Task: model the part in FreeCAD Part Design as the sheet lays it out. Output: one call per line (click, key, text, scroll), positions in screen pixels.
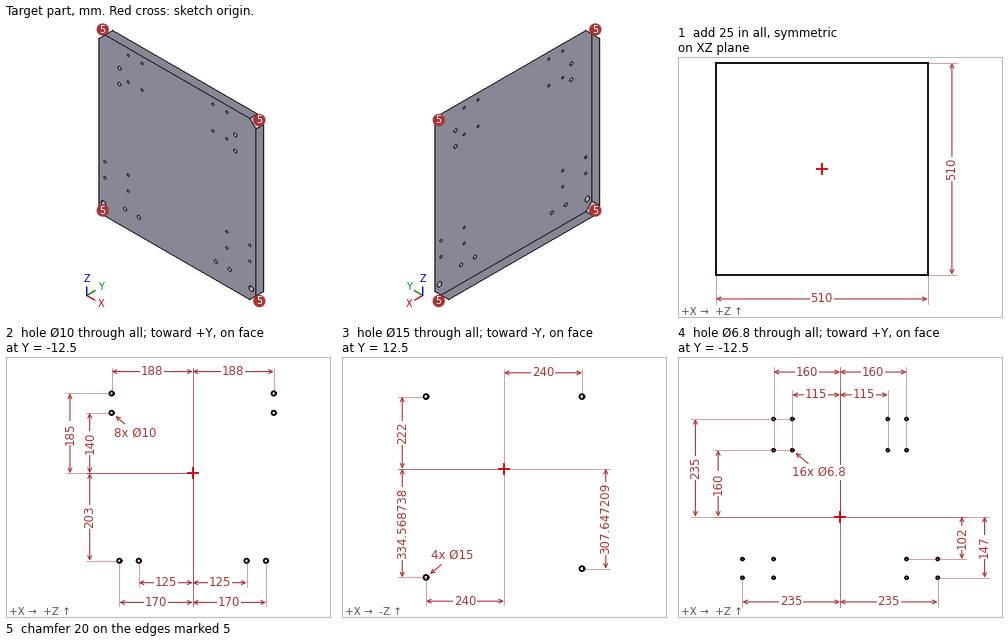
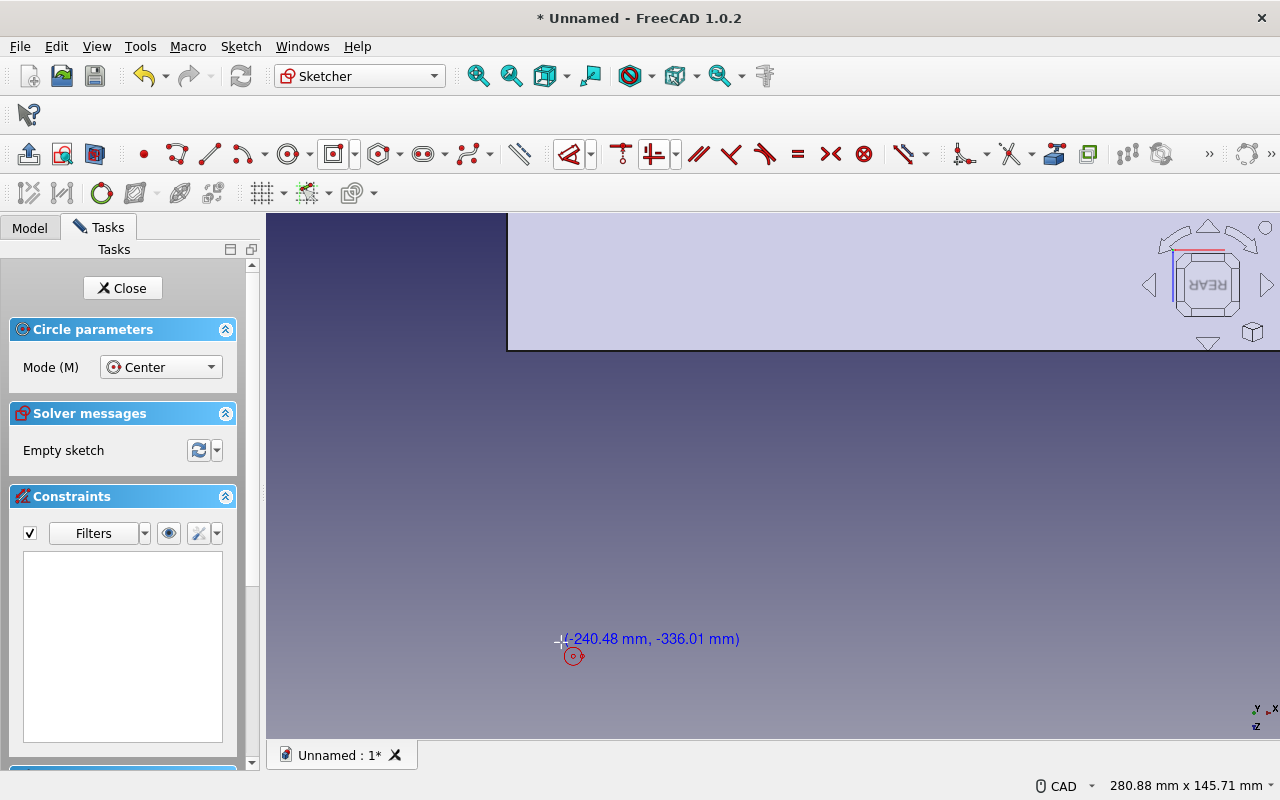
scroll(561, 643, down, 9)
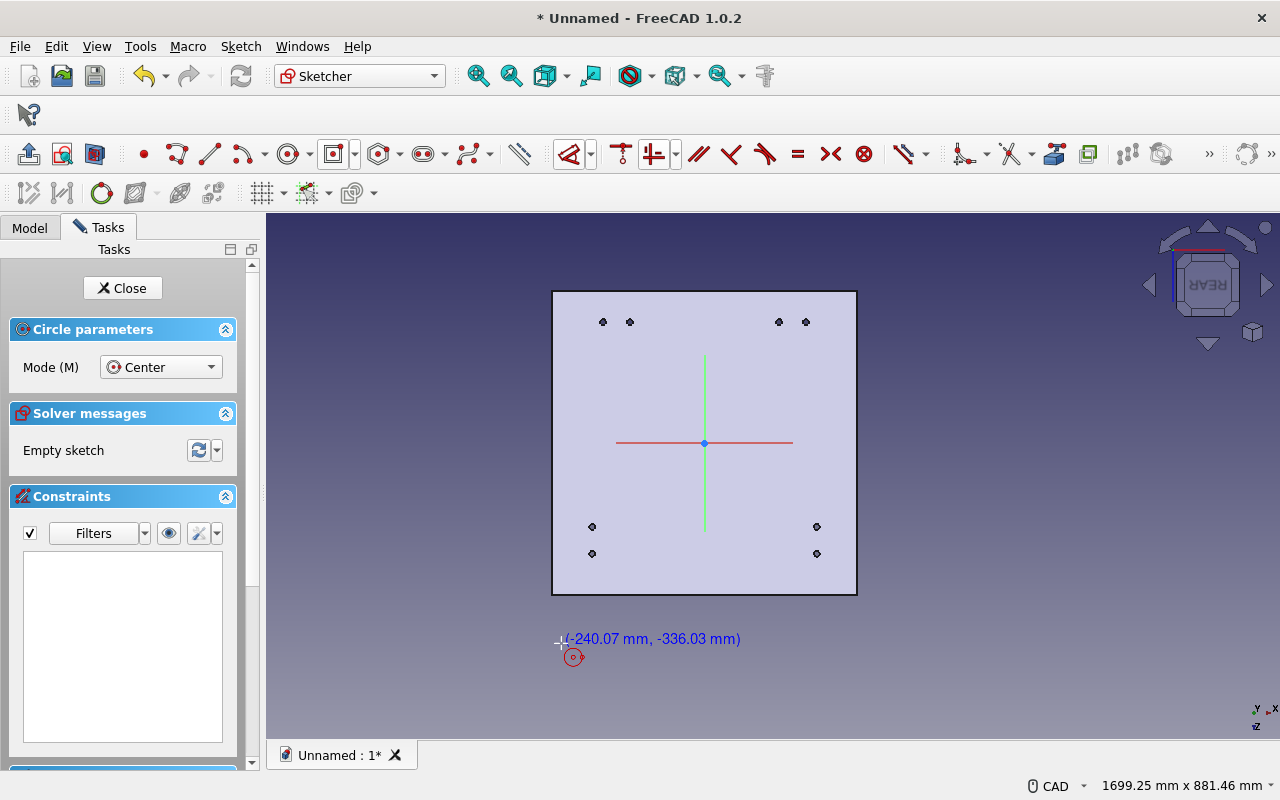
click(561, 643)
move(564, 640)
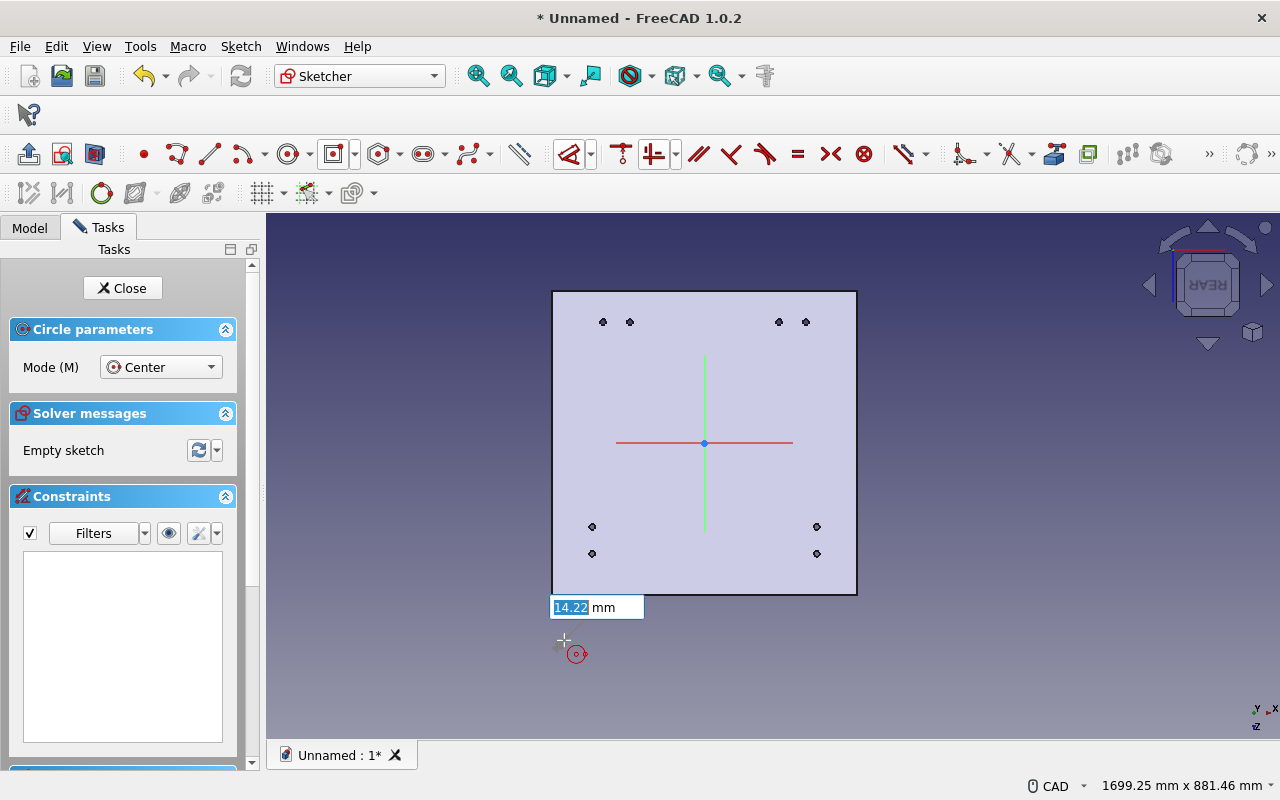
text(15)
key(Return)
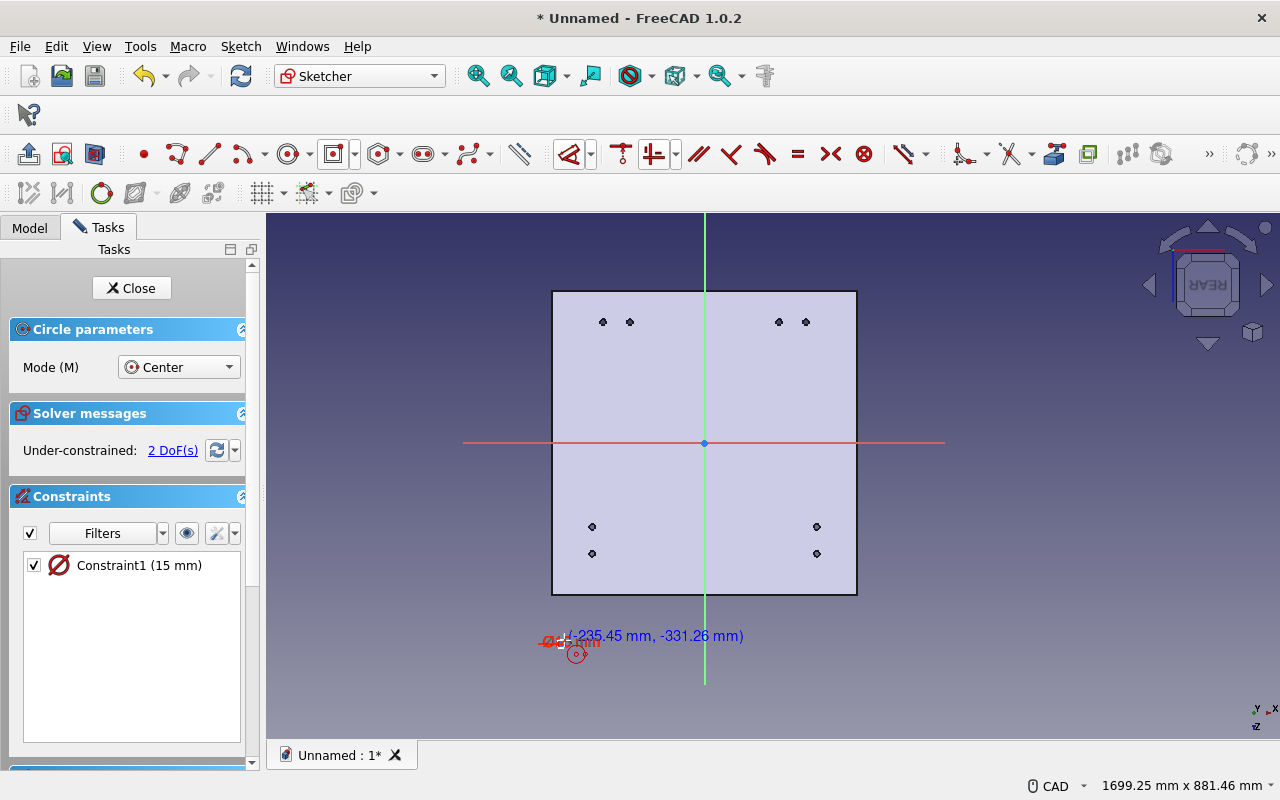
scroll(561, 311, up, 9)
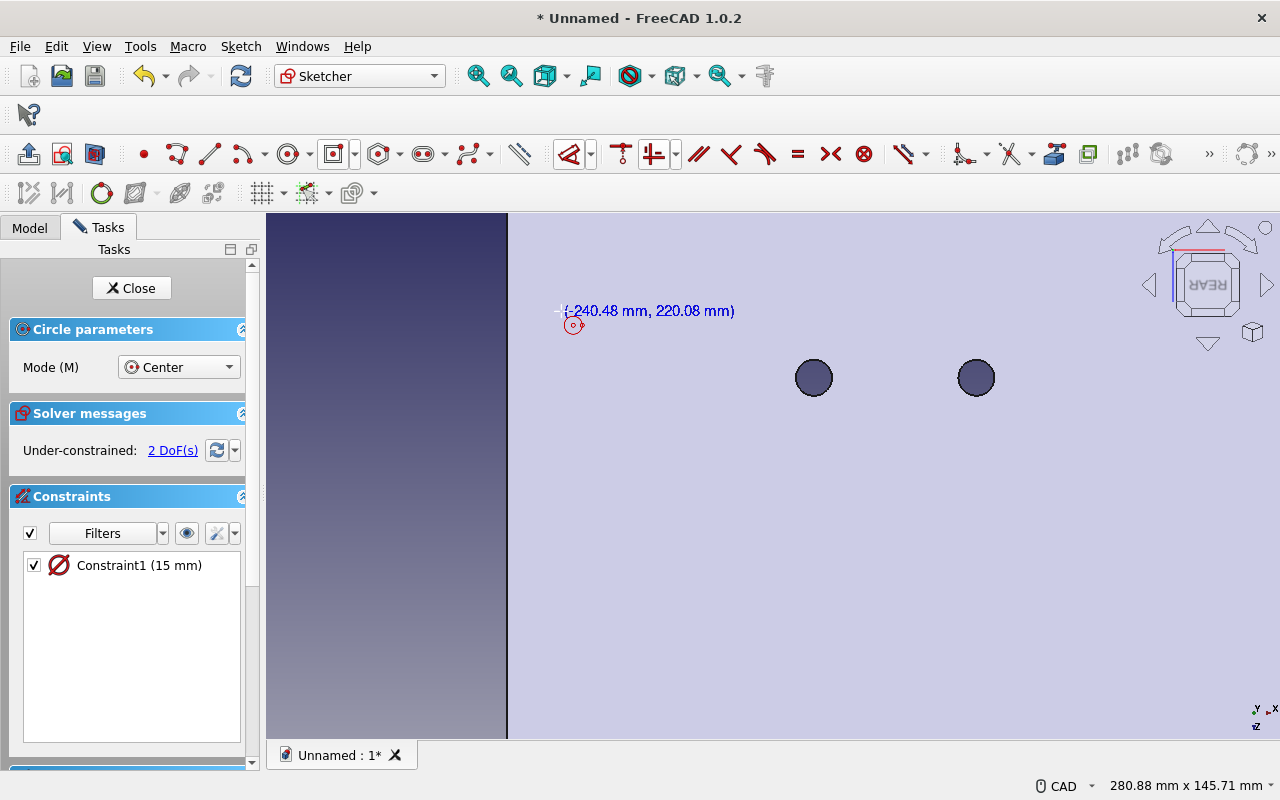
scroll(561, 310, down, 9)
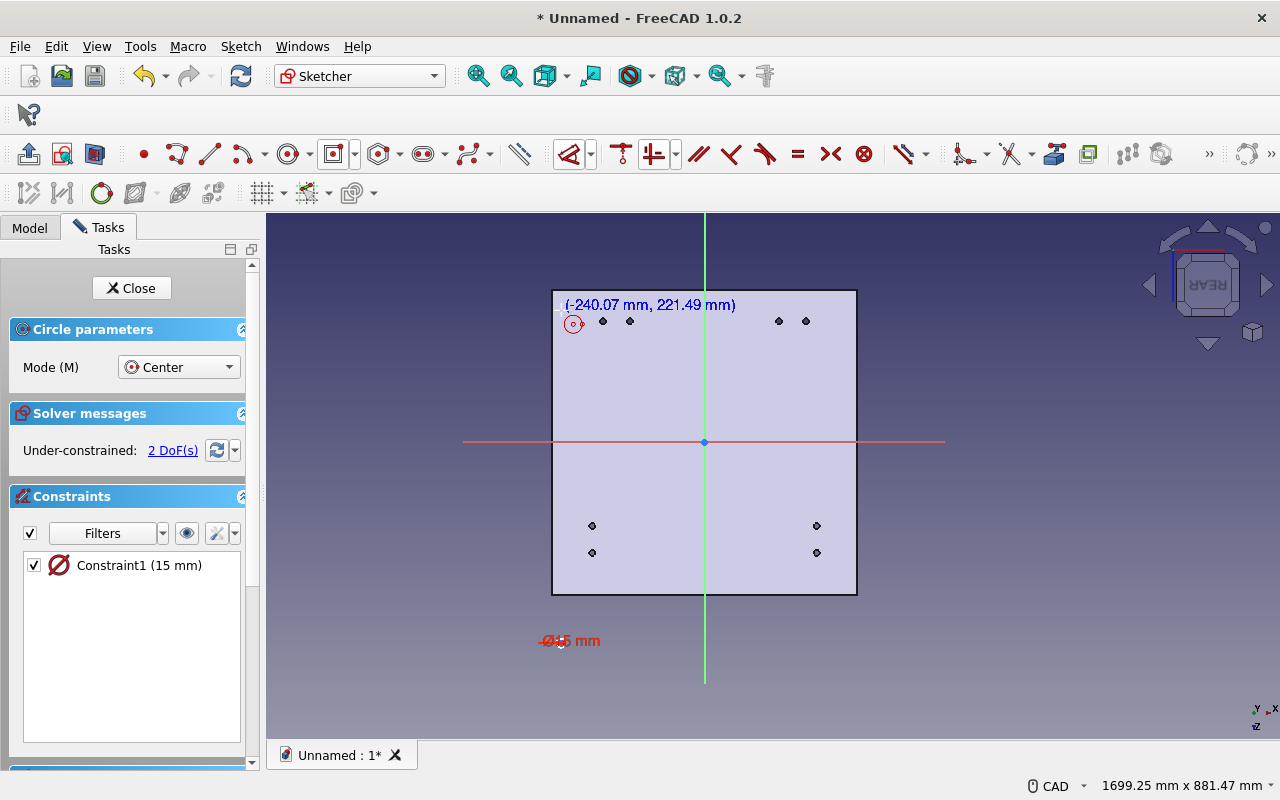
click(561, 310)
move(564, 307)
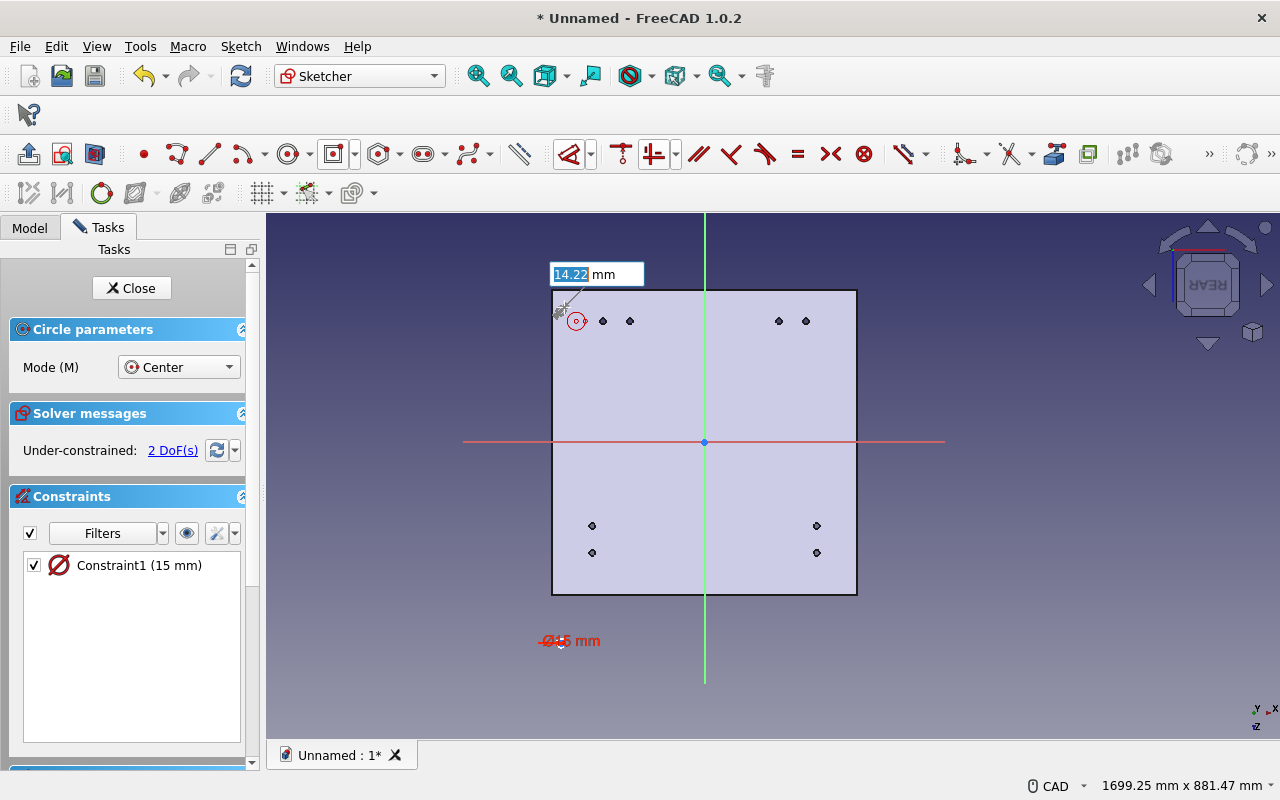
text(15)
key(Return)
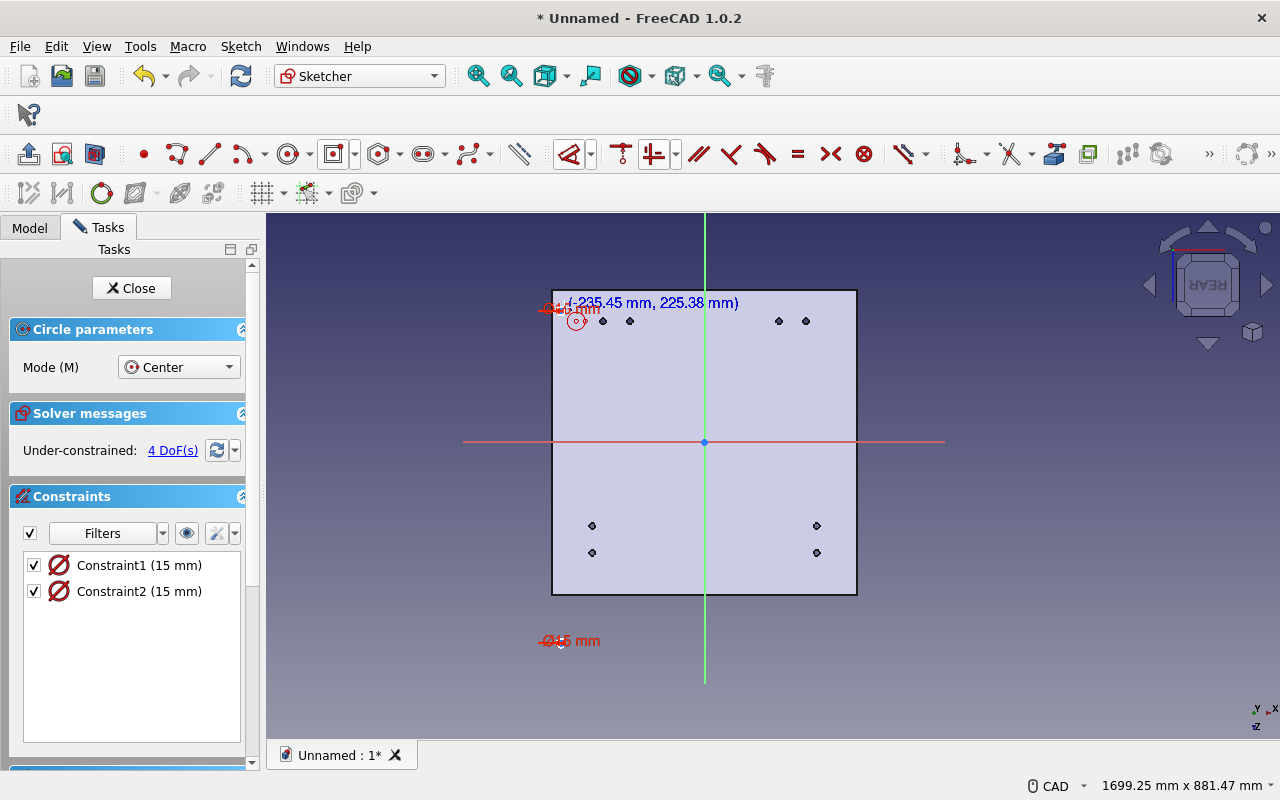
scroll(848, 310, up, 9)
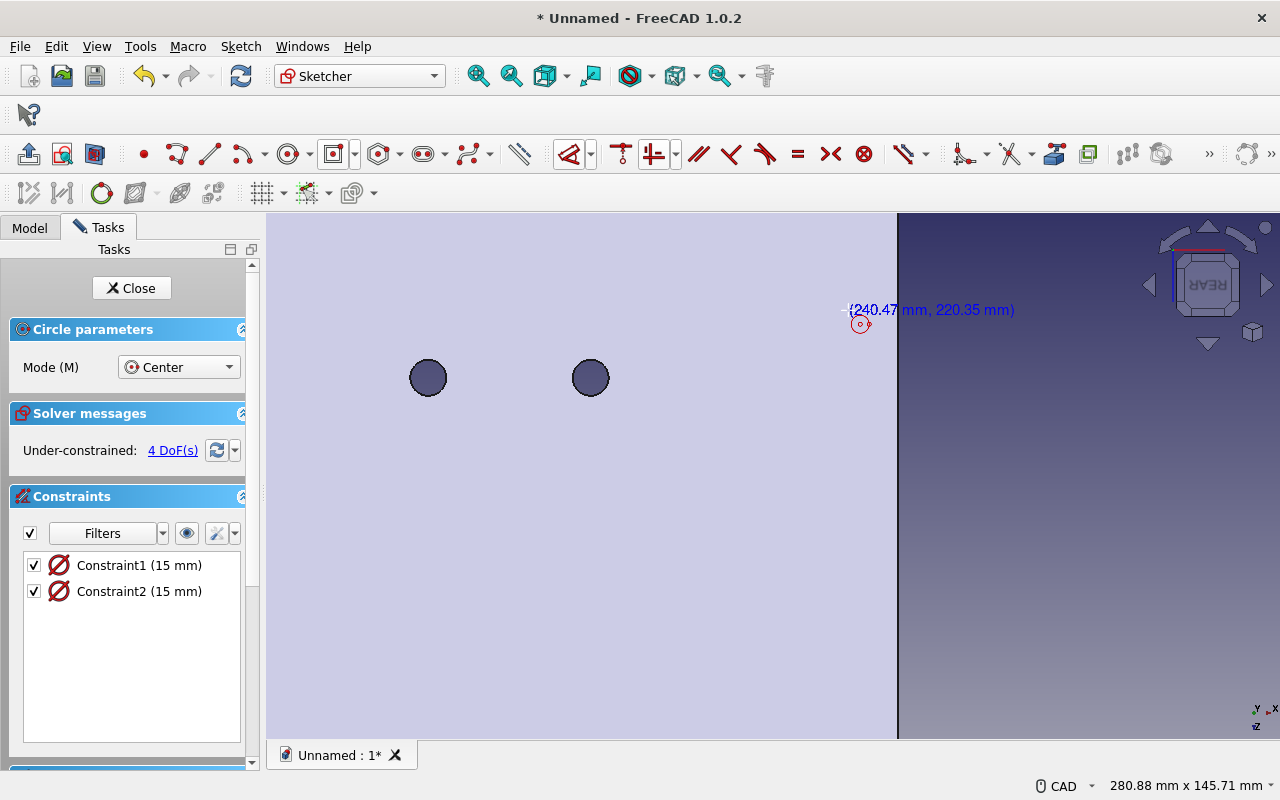
scroll(849, 310, down, 9)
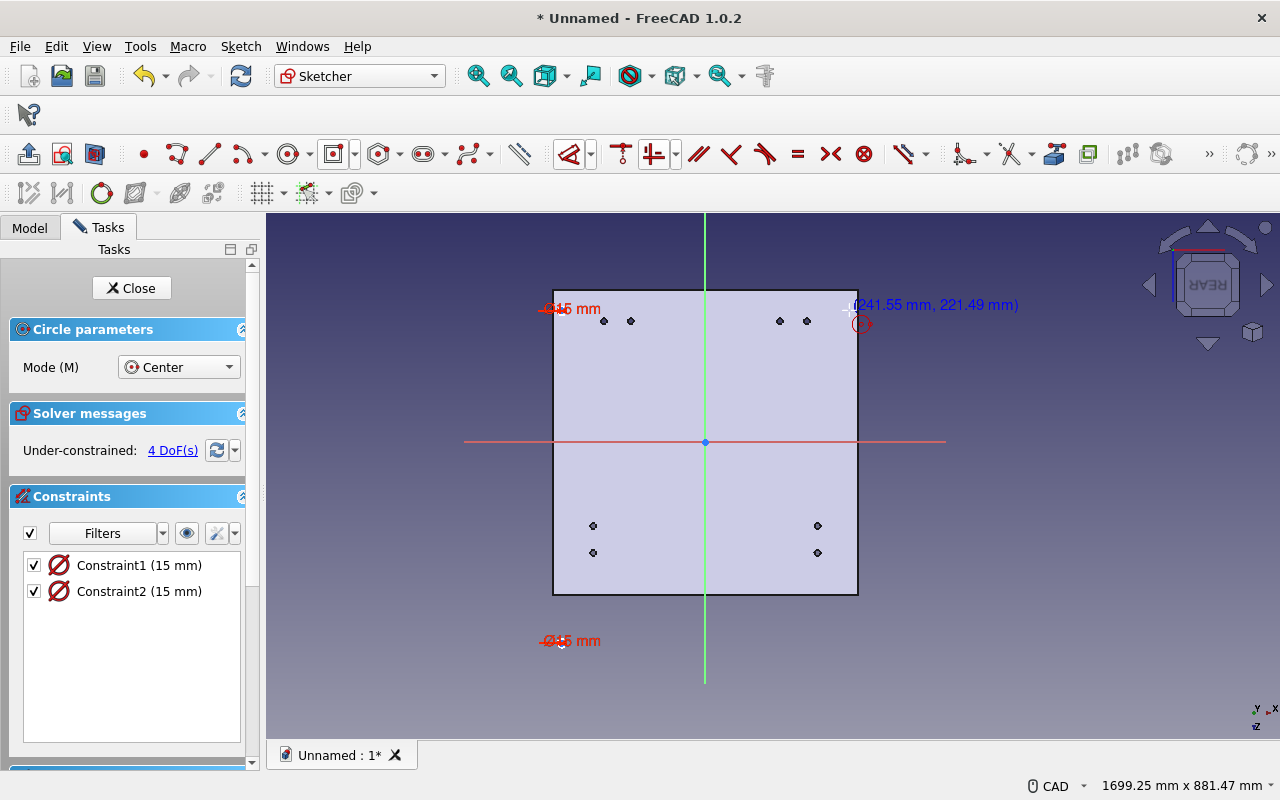
click(849, 310)
move(852, 307)